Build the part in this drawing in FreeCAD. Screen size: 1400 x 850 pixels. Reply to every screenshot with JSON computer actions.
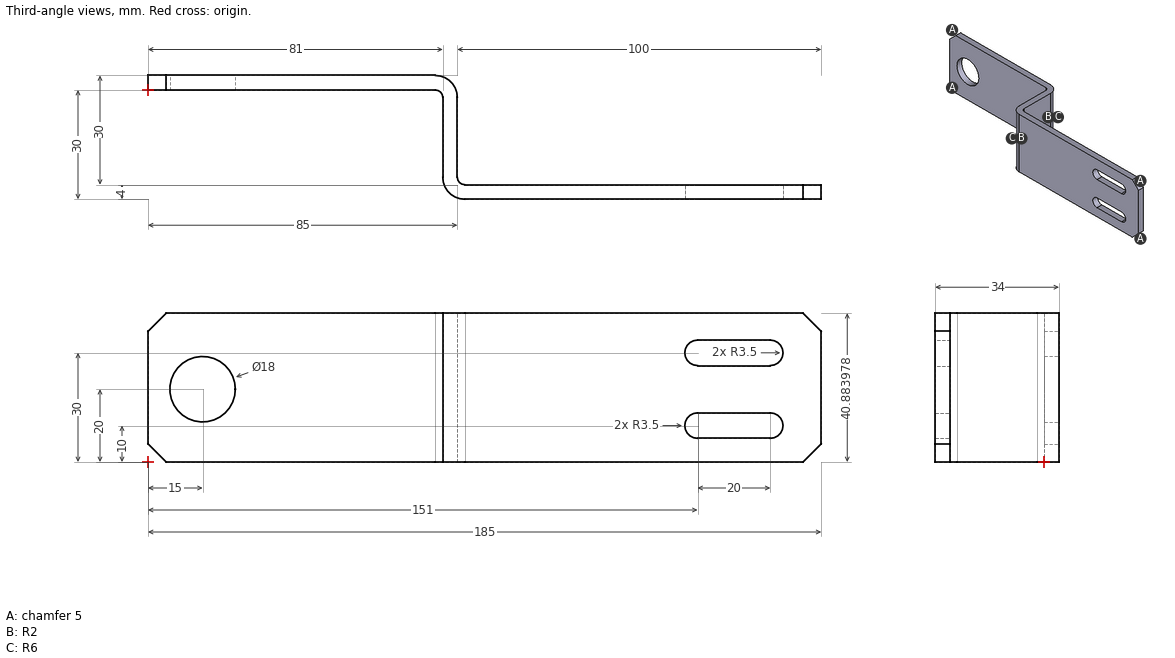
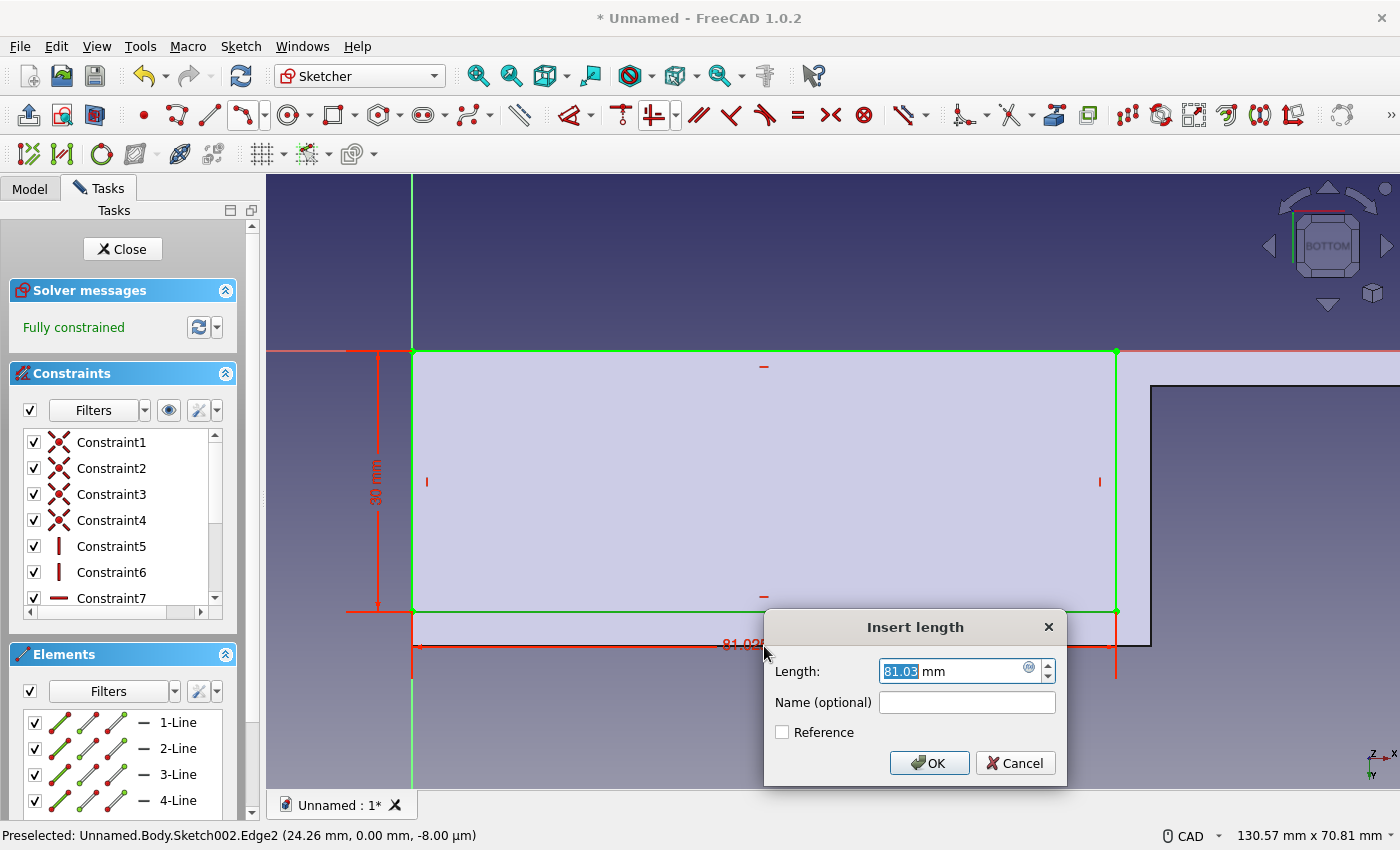
{"action": "type", "text": "81"}
{"action": "key", "text": "Return"}
{"action": "key", "text": "Escape"}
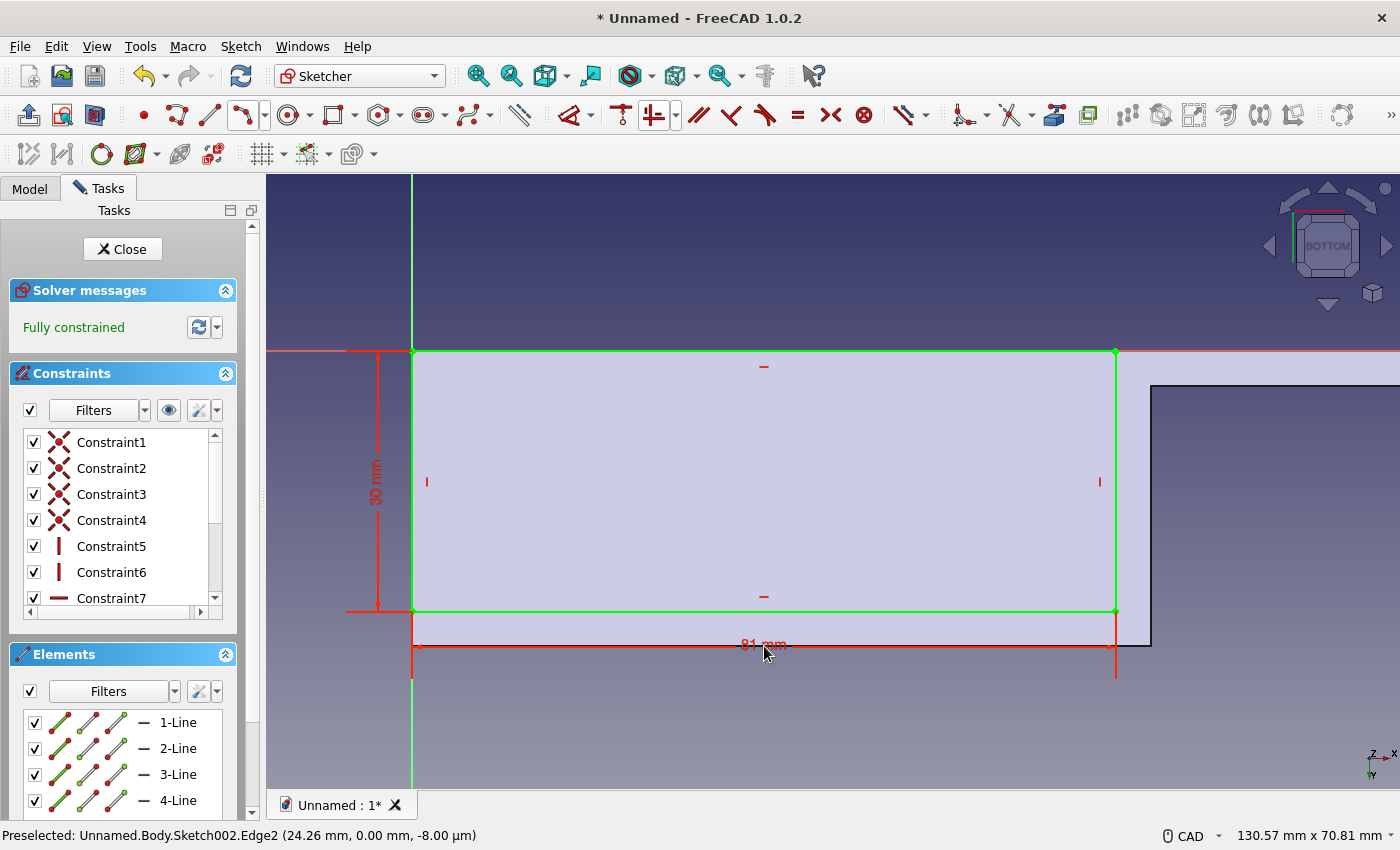
{"action": "left_click", "coordinate": [123, 249]}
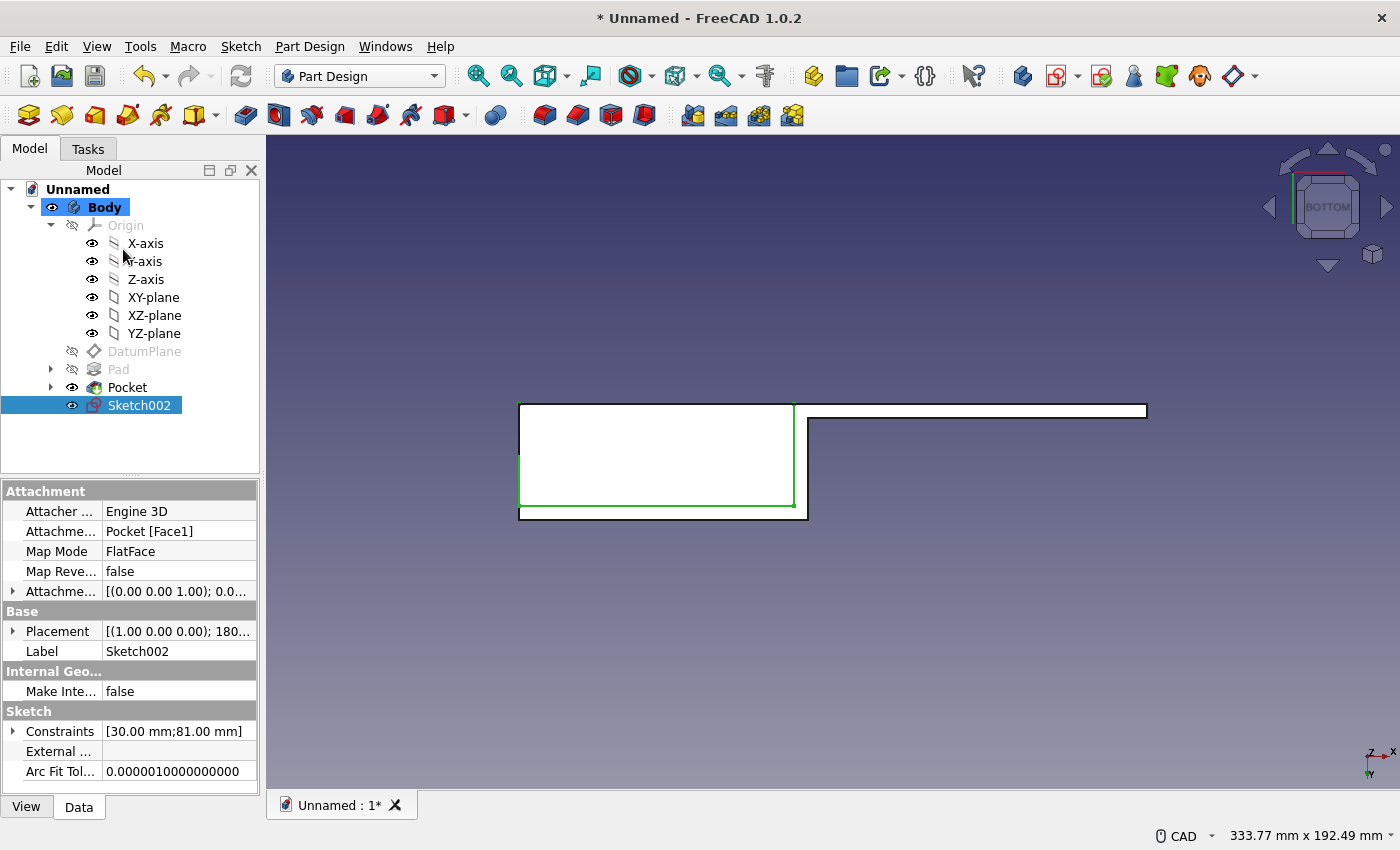
{"action": "left_click", "coordinate": [246, 116]}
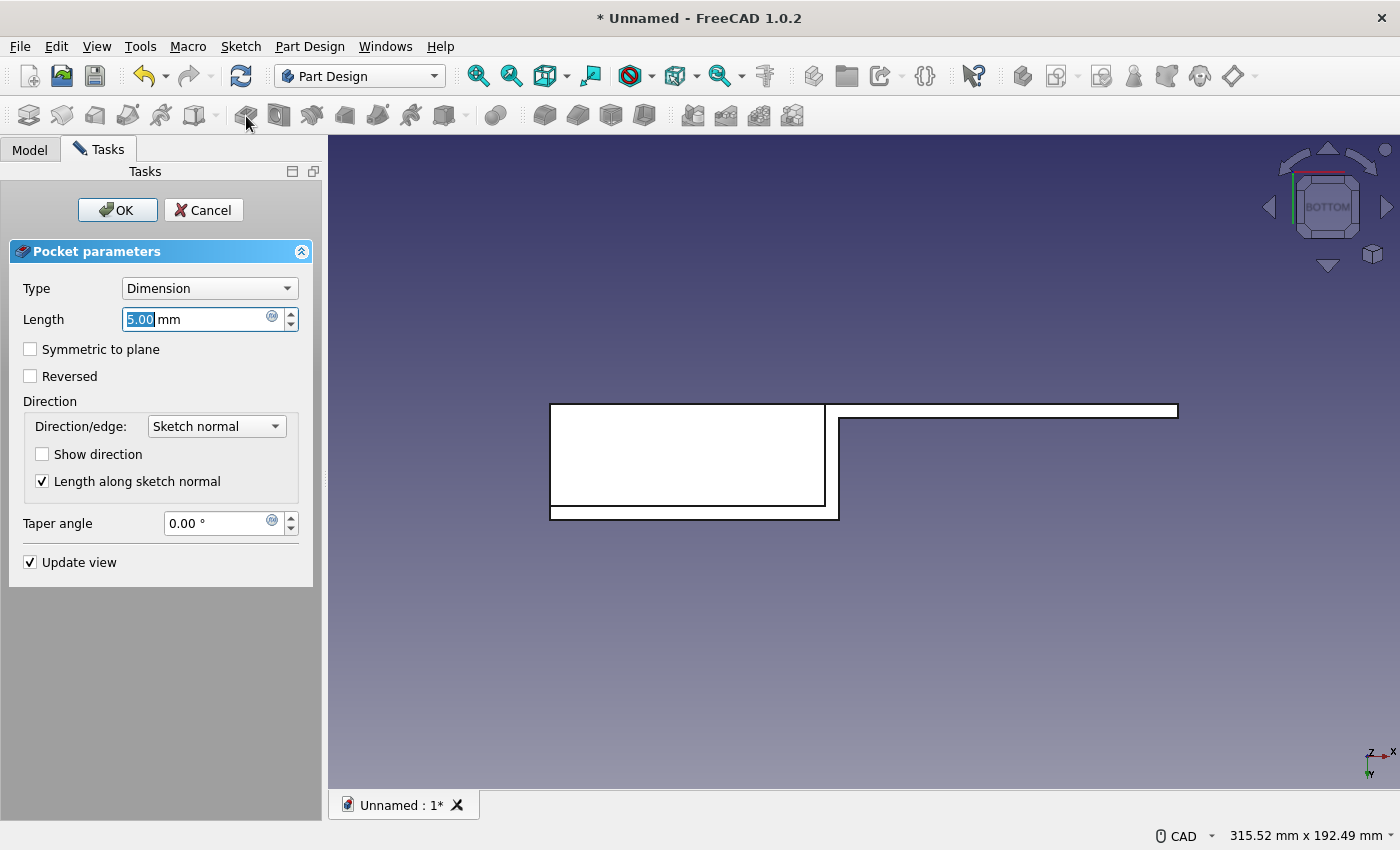
{"action": "left_click", "coordinate": [210, 288]}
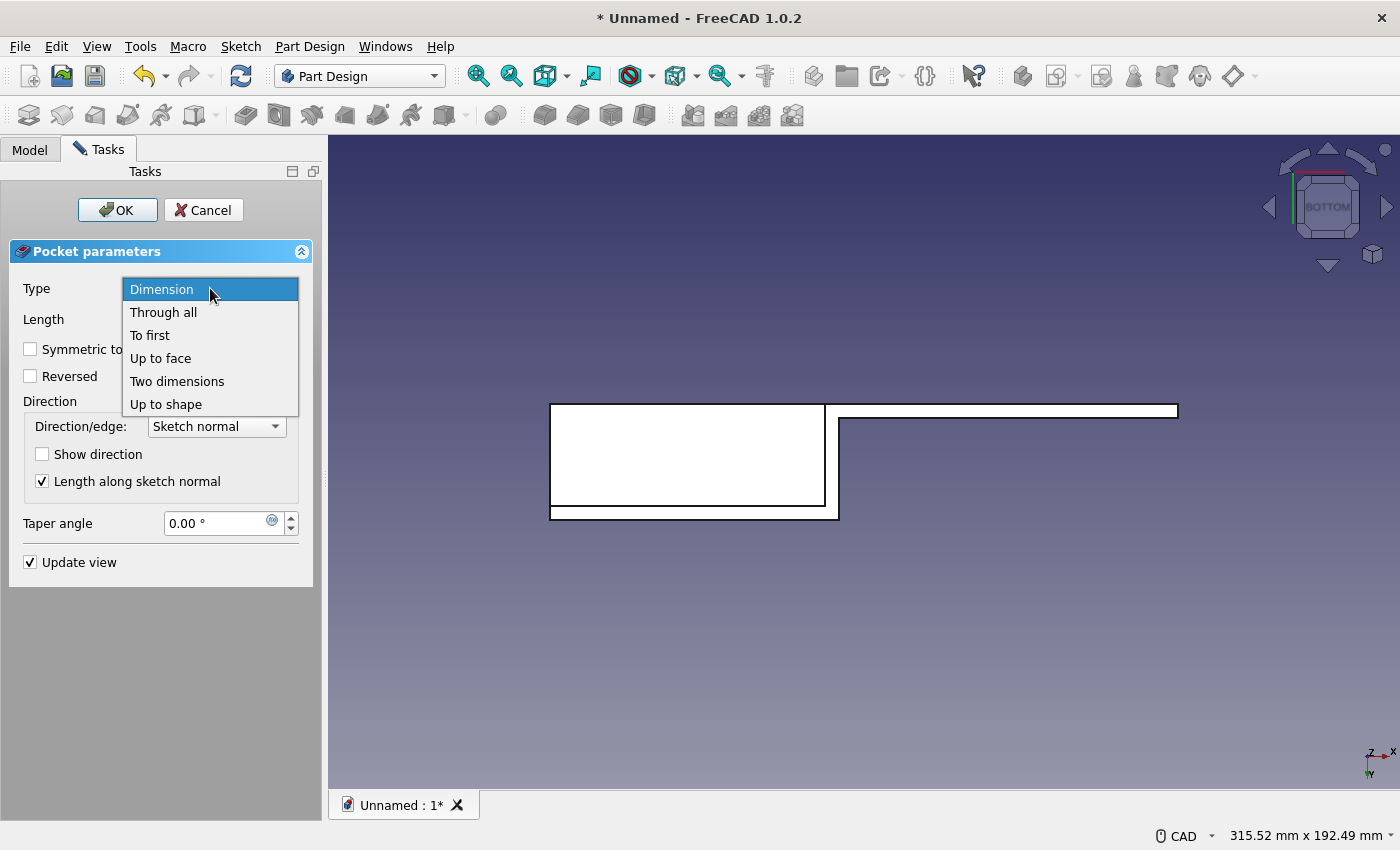
{"action": "left_click", "coordinate": [208, 312]}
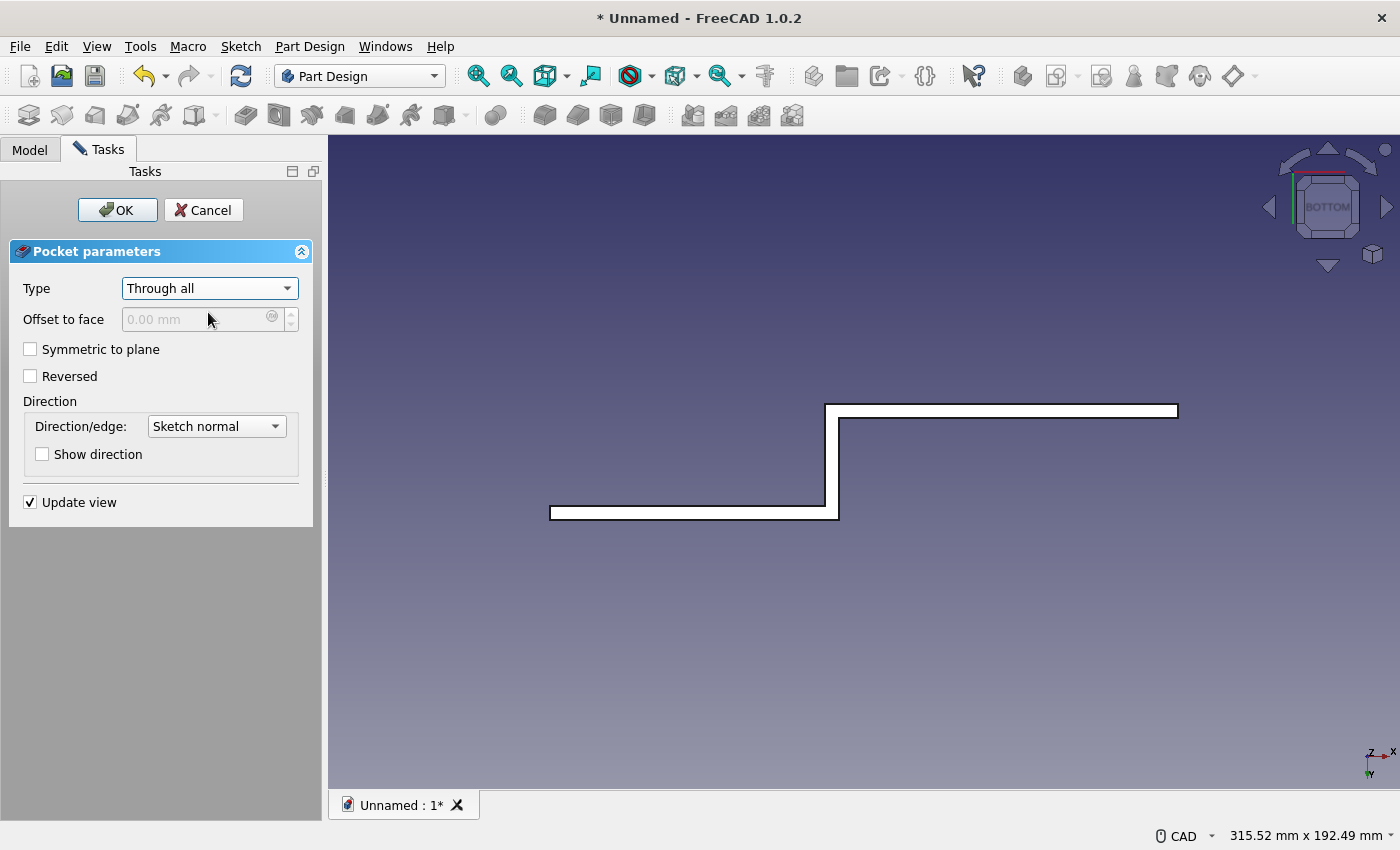
{"action": "left_click", "coordinate": [118, 210]}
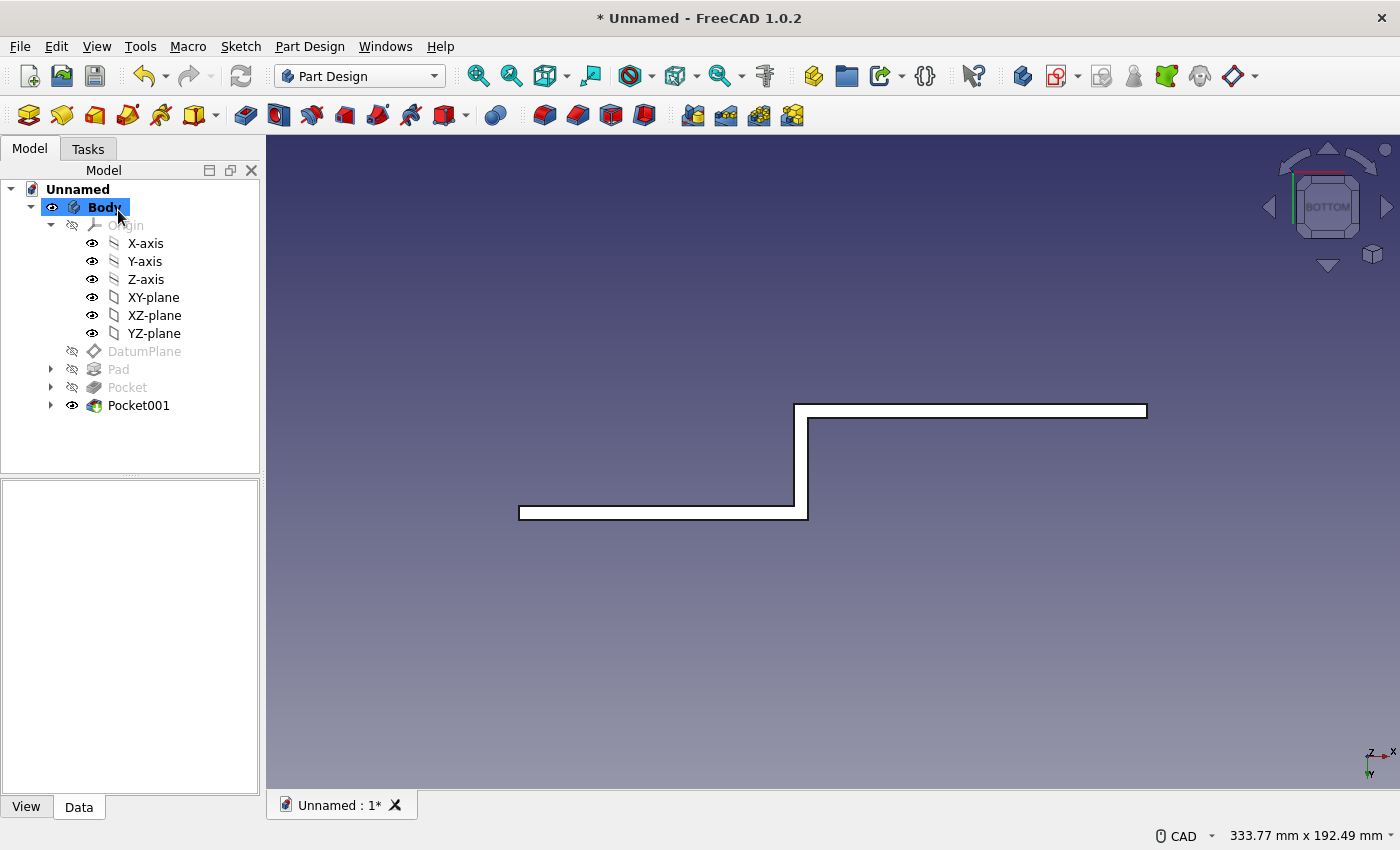
{"action": "key", "text": "0"}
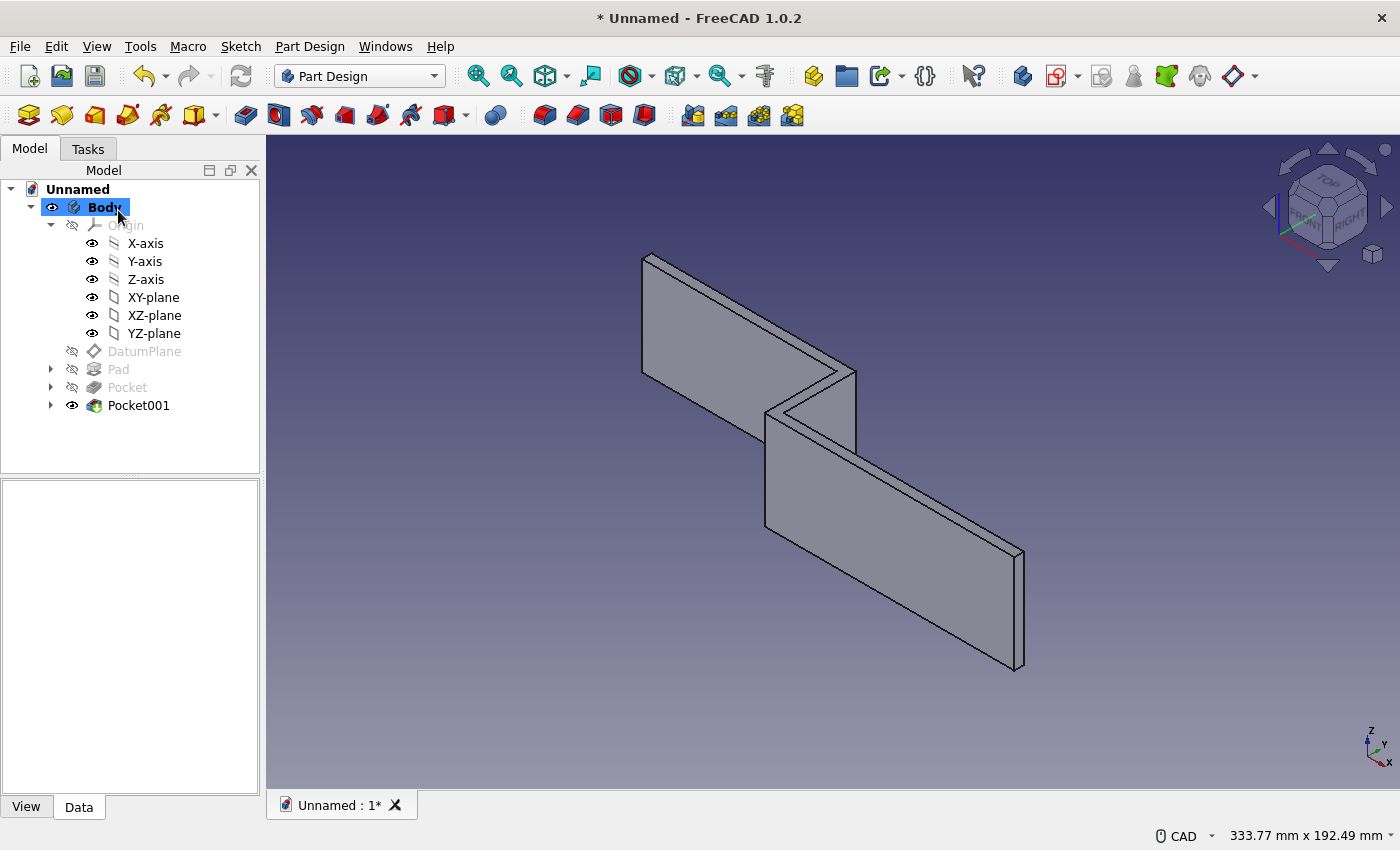
{"action": "left_click", "coordinate": [961, 582]}